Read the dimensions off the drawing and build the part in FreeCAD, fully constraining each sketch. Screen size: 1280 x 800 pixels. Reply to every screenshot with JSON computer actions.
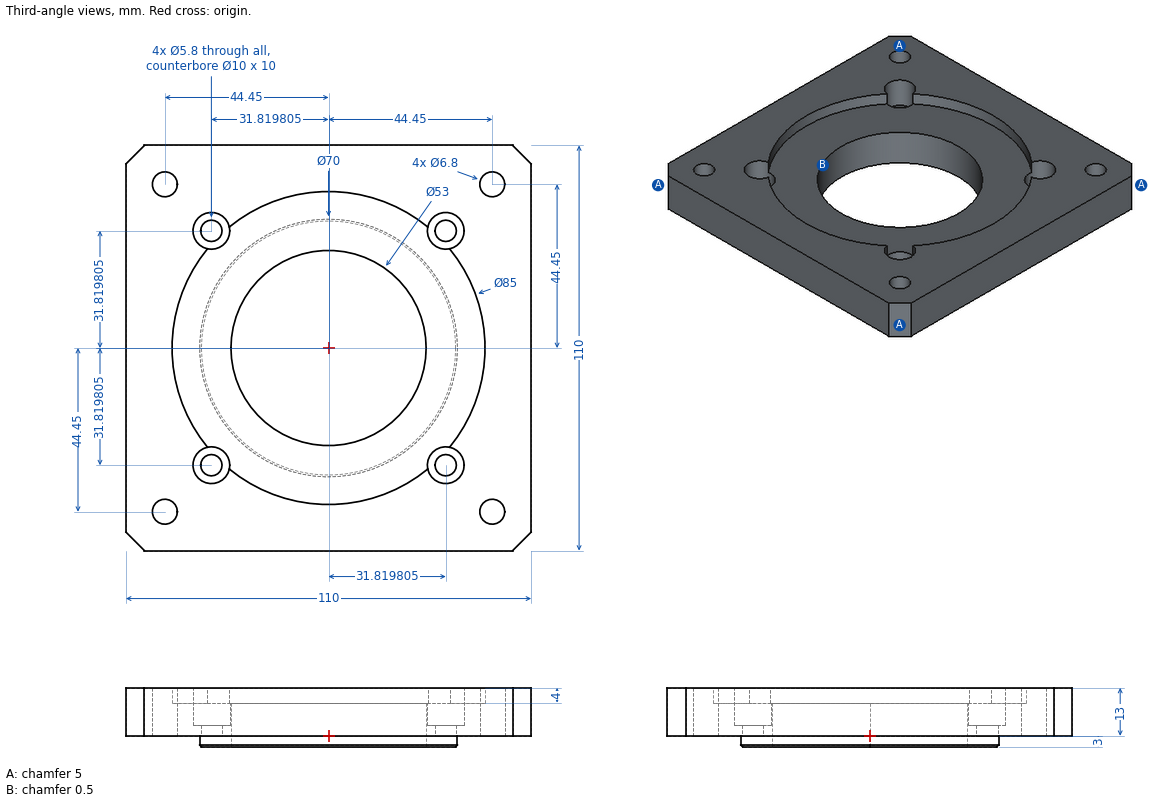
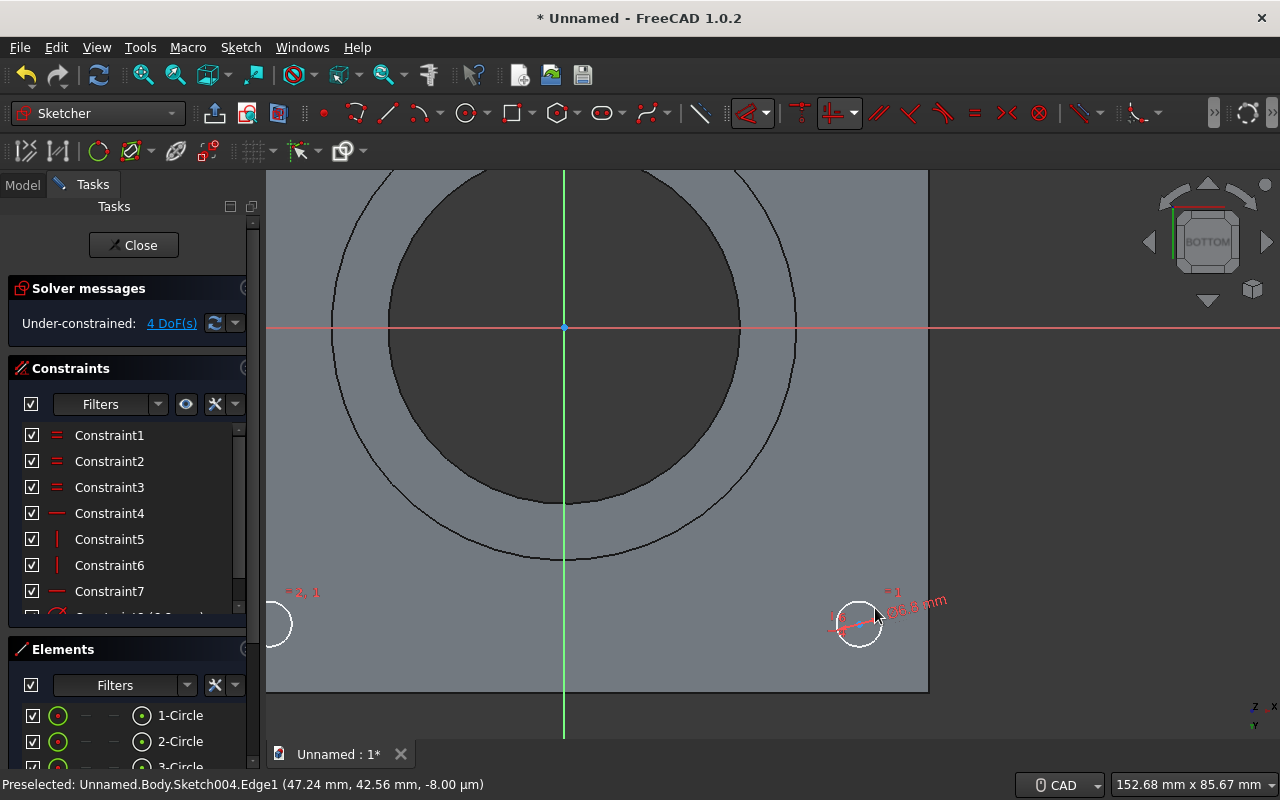
{"action": "left_click", "coordinate": [859, 624]}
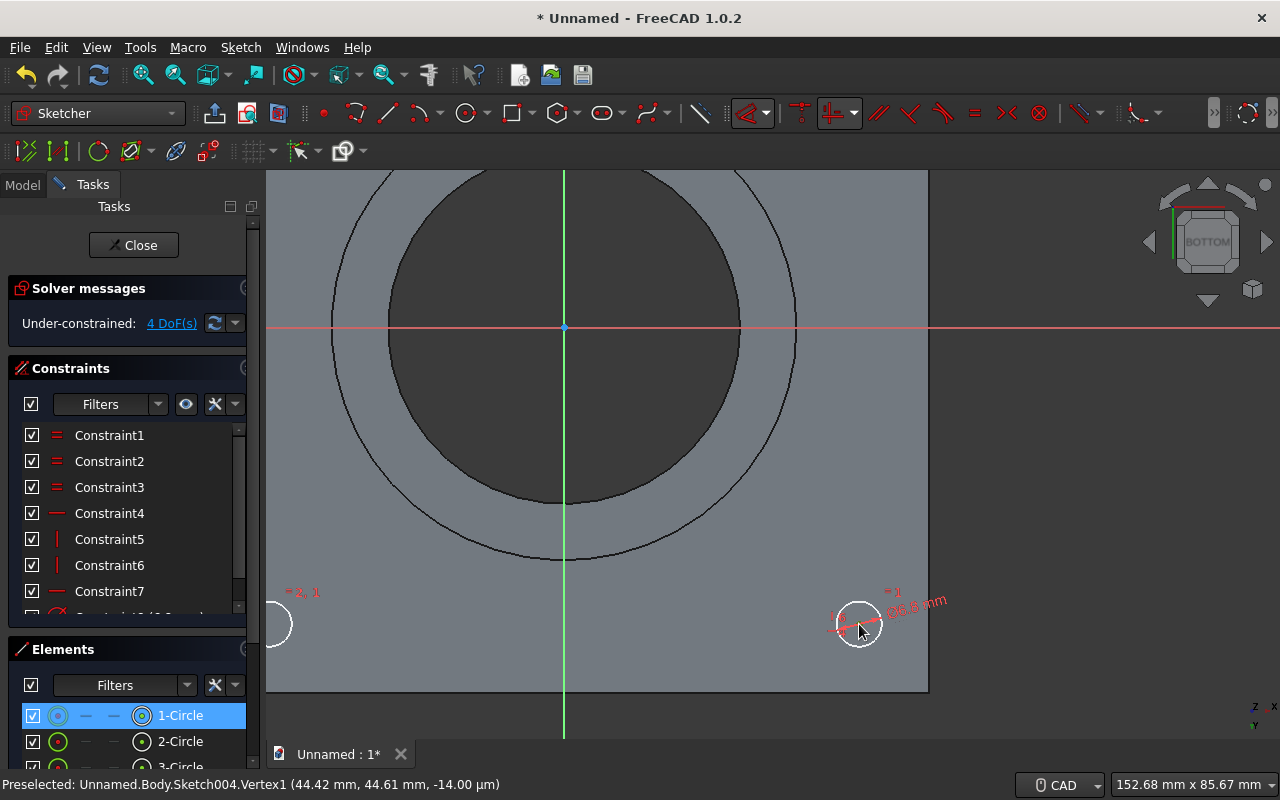
{"action": "left_click", "coordinate": [768, 114]}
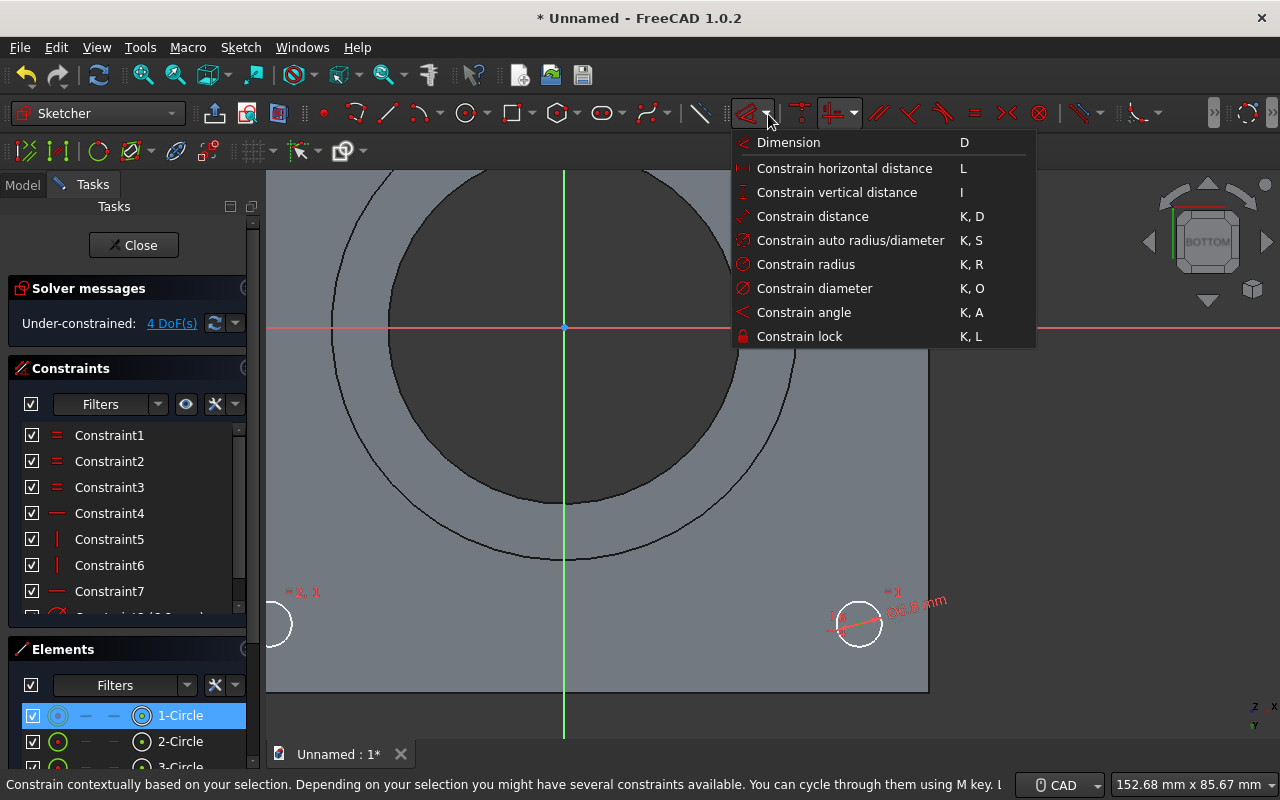
{"action": "left_click", "coordinate": [884, 168]}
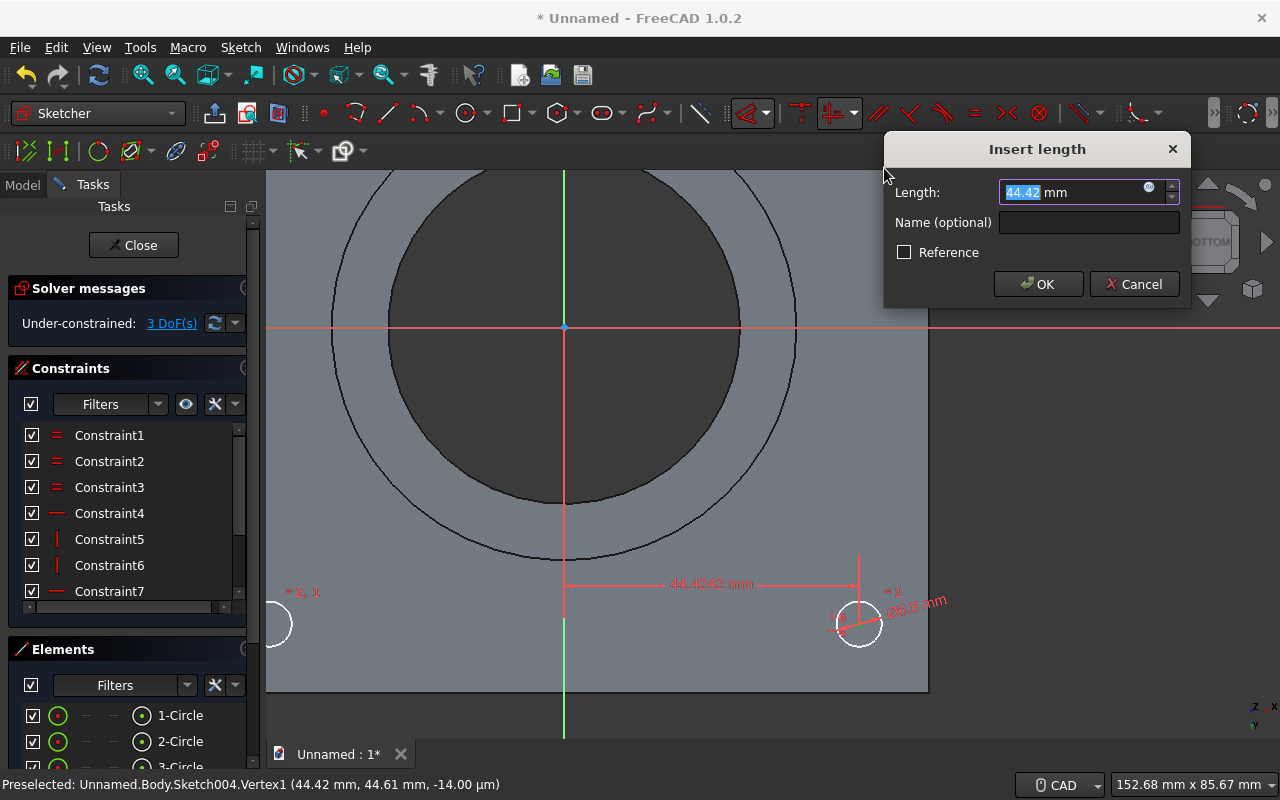
{"action": "type", "text": "44.45"}
{"action": "key", "text": "Return"}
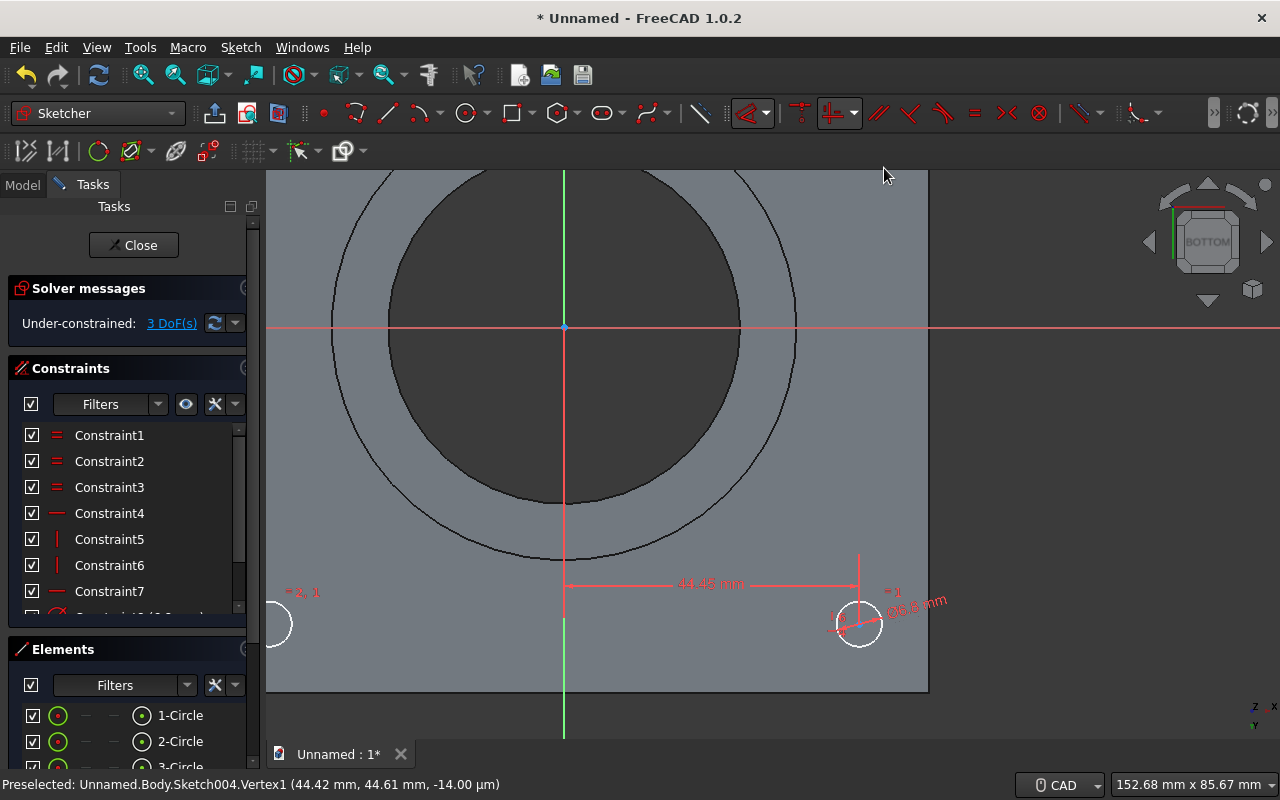
{"action": "left_click", "coordinate": [859, 624]}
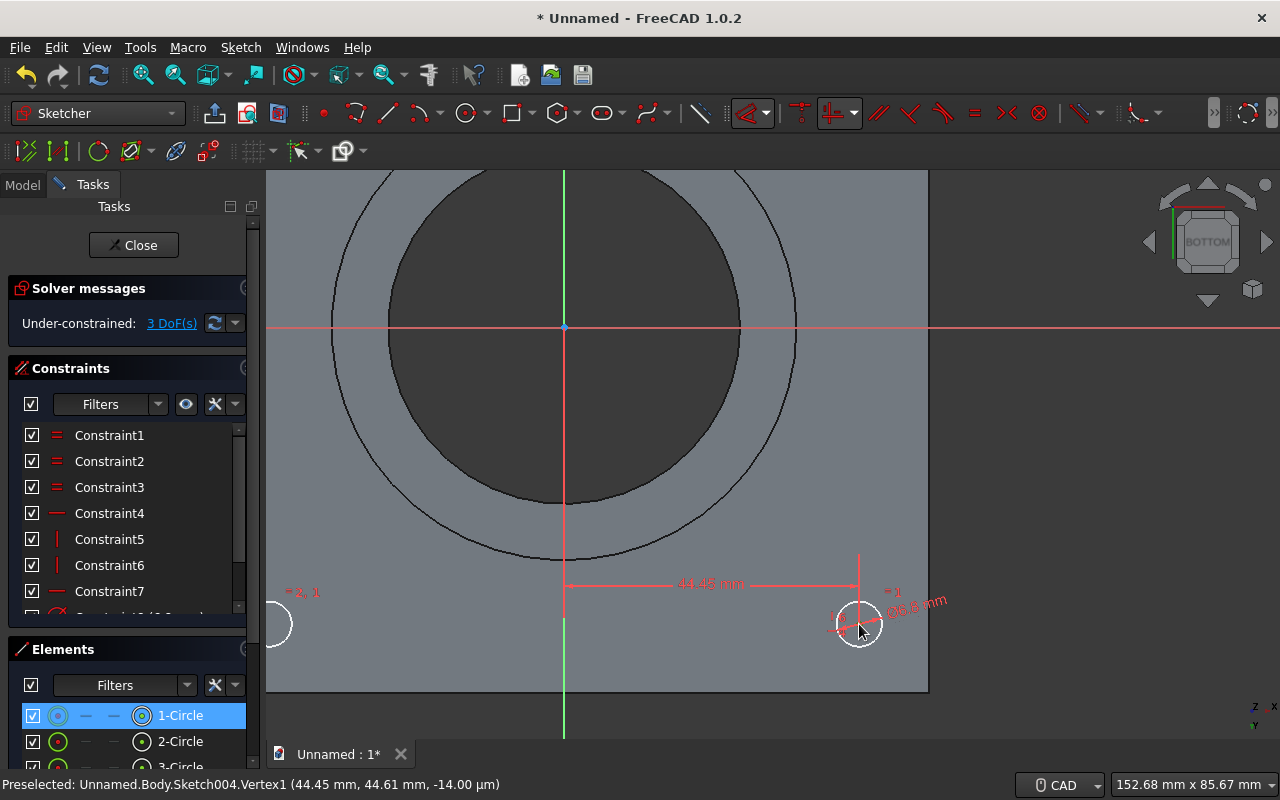
{"action": "key", "text": "i"}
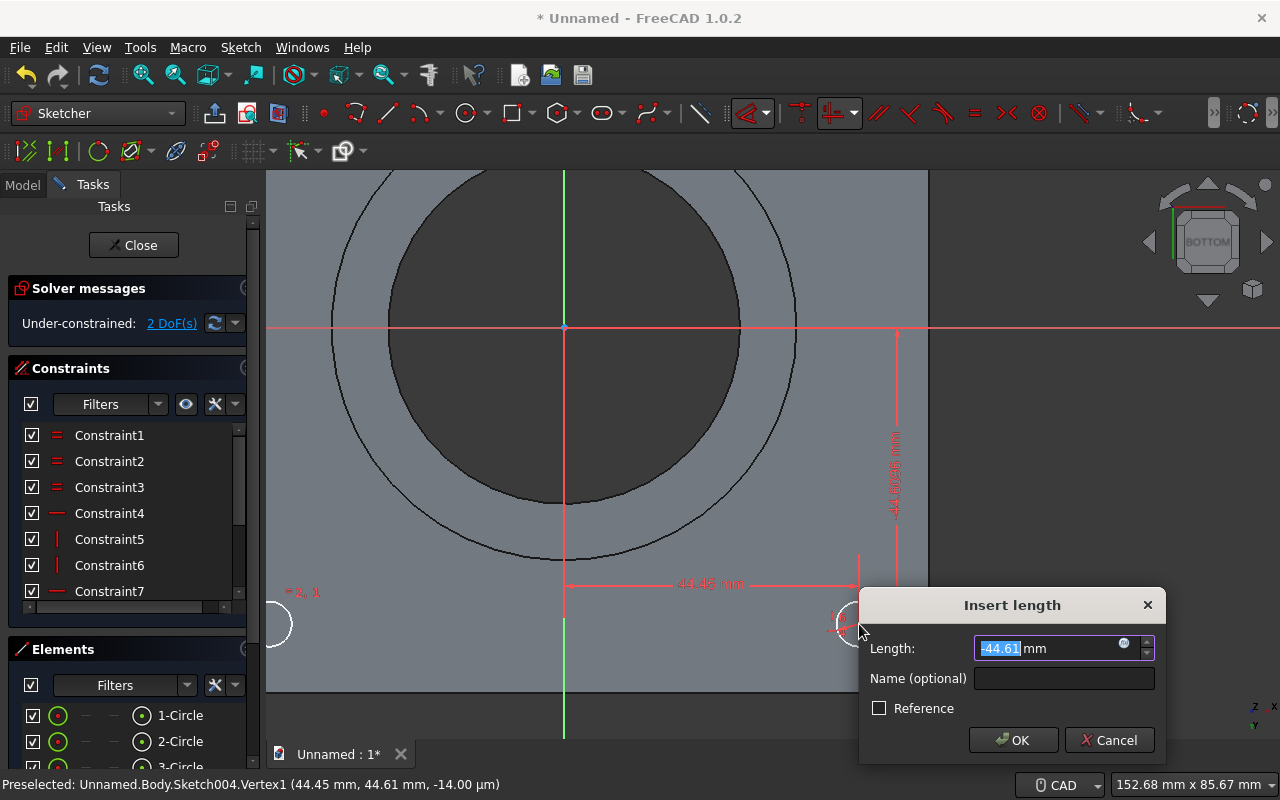
{"action": "type", "text": "-44.45"}
{"action": "key", "text": "Return"}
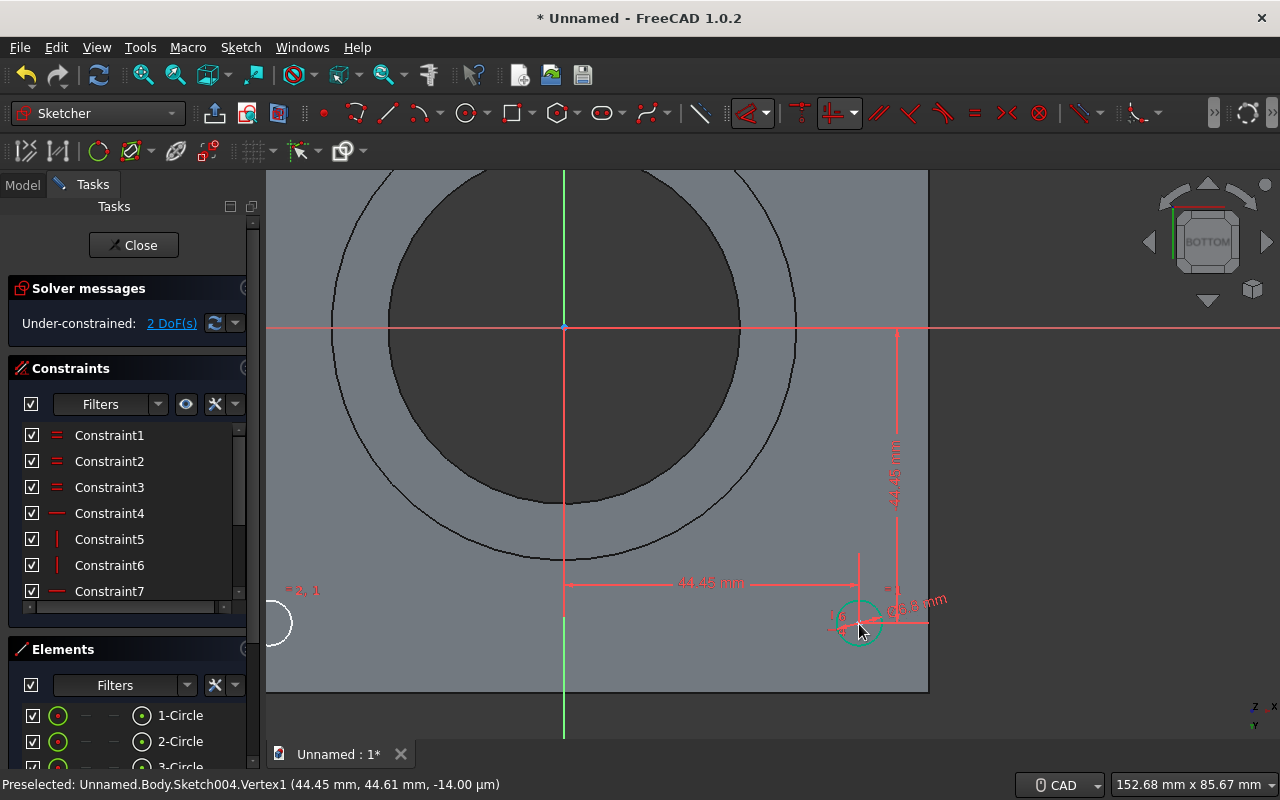
{"action": "scroll", "coordinate": [875, 609], "scroll_direction": "down", "scroll_amount": 3}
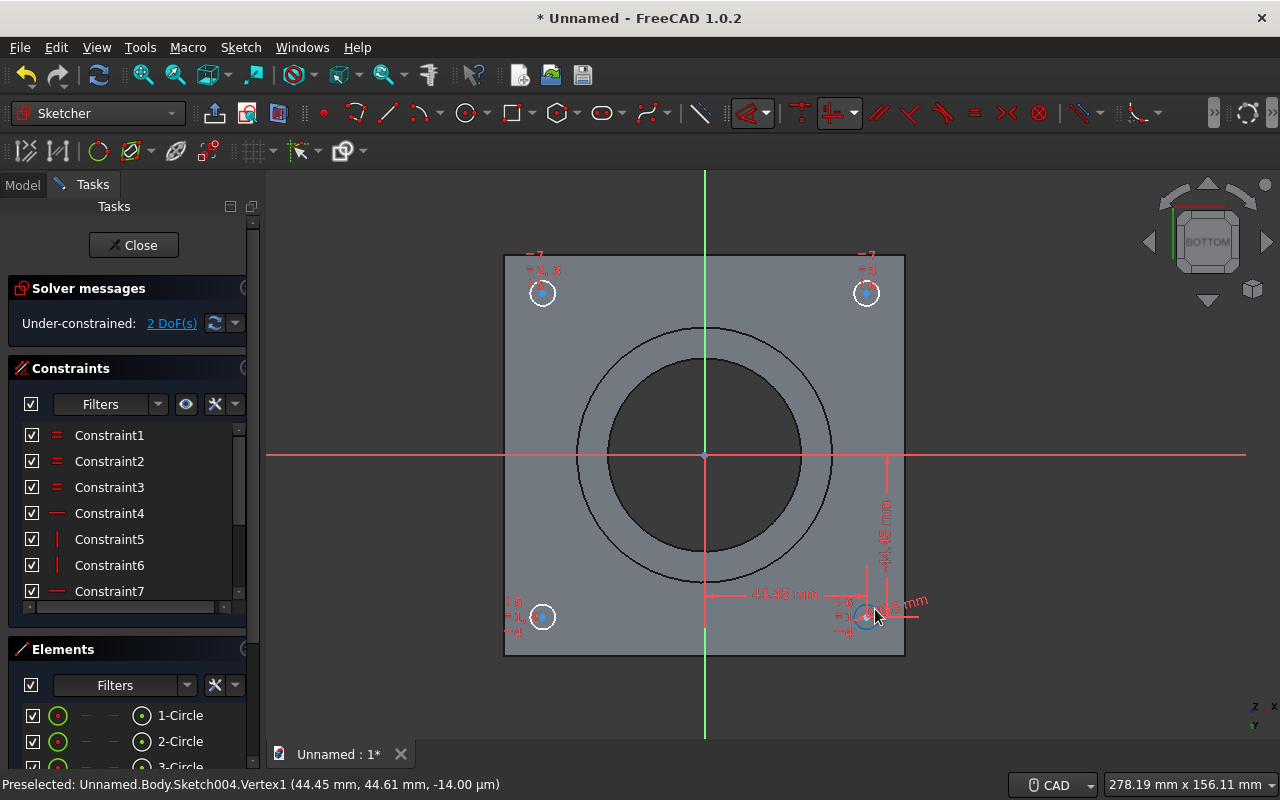
{"action": "left_click", "coordinate": [543, 617]}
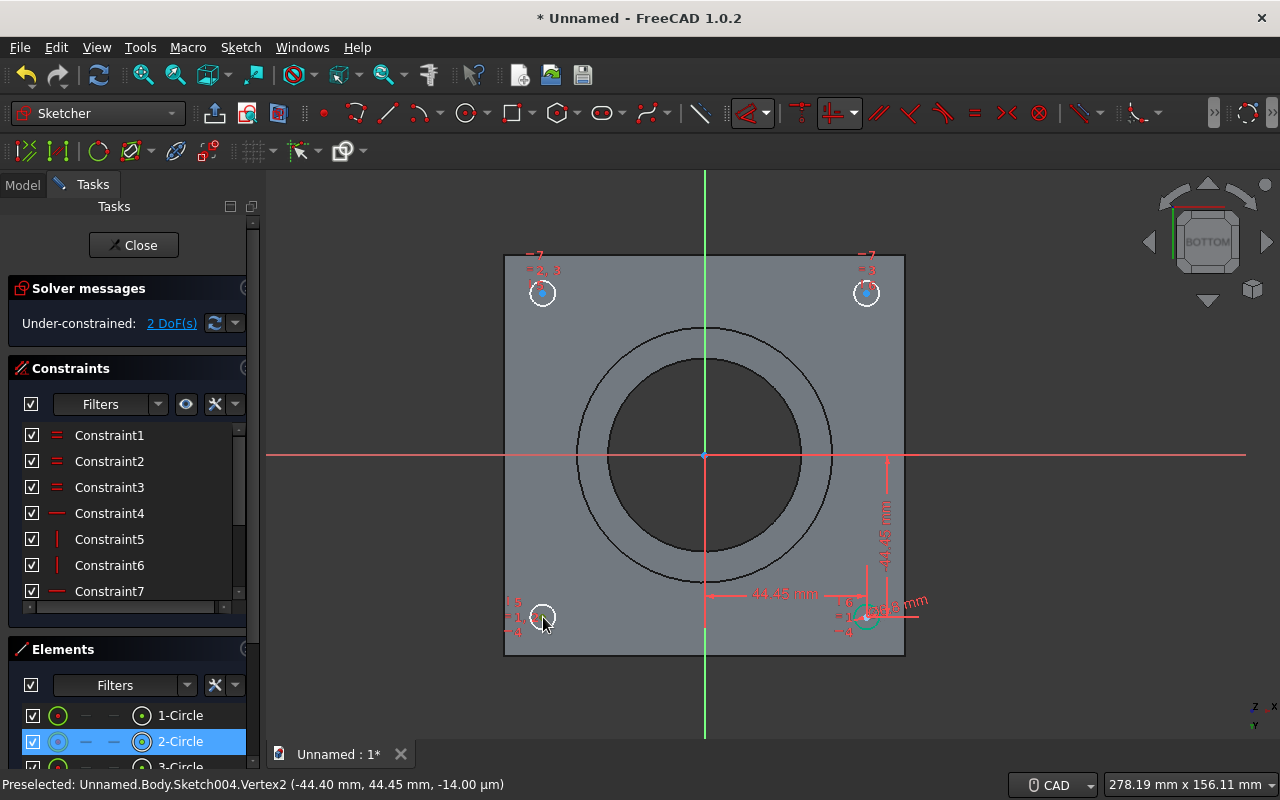
{"action": "key", "text": "l"}